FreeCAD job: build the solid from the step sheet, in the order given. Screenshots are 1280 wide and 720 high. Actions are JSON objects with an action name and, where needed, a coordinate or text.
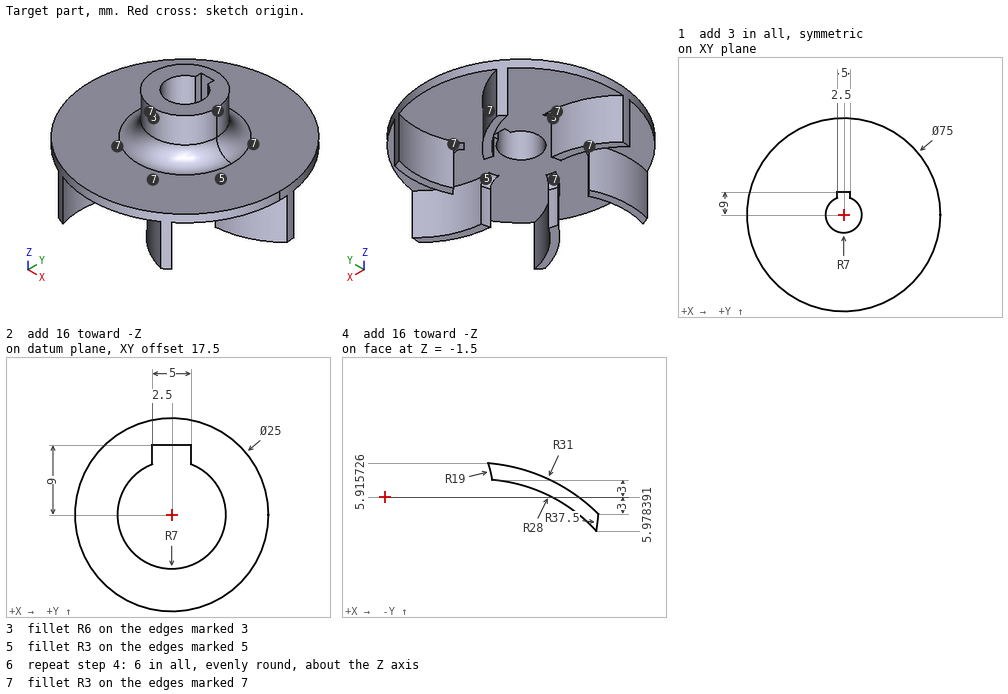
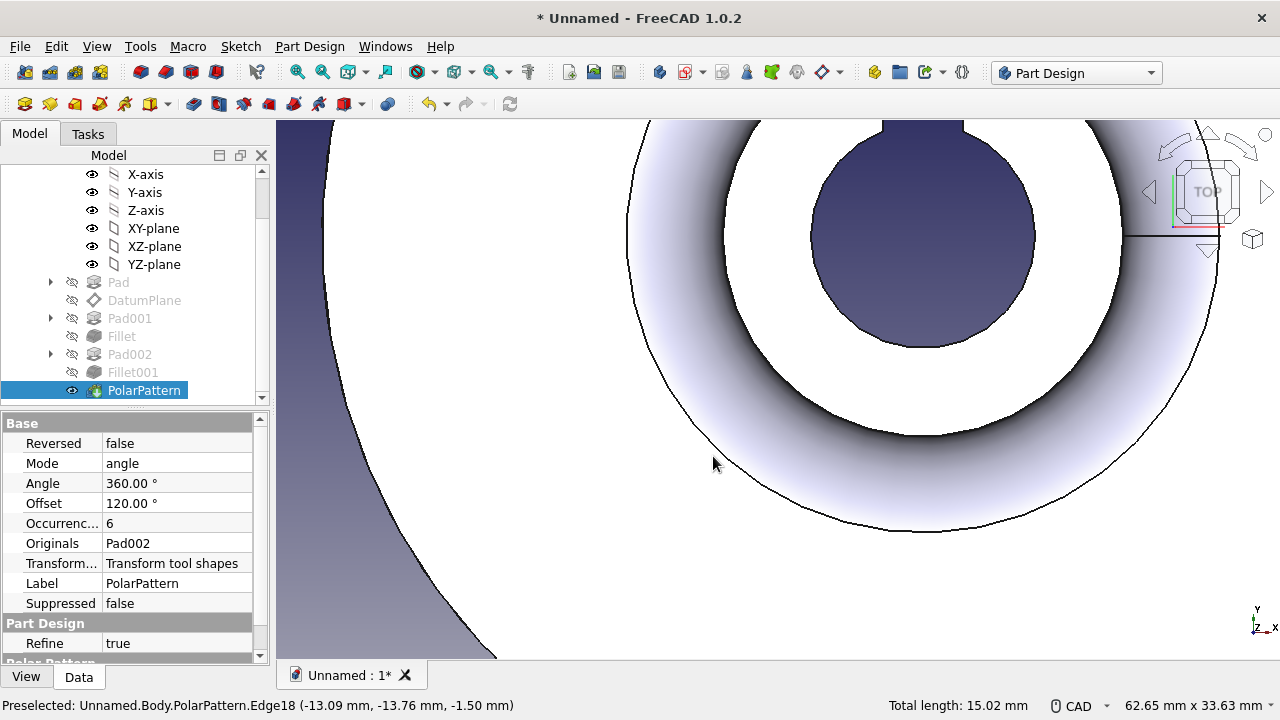
{"action": "left_click", "coordinate": [141, 72]}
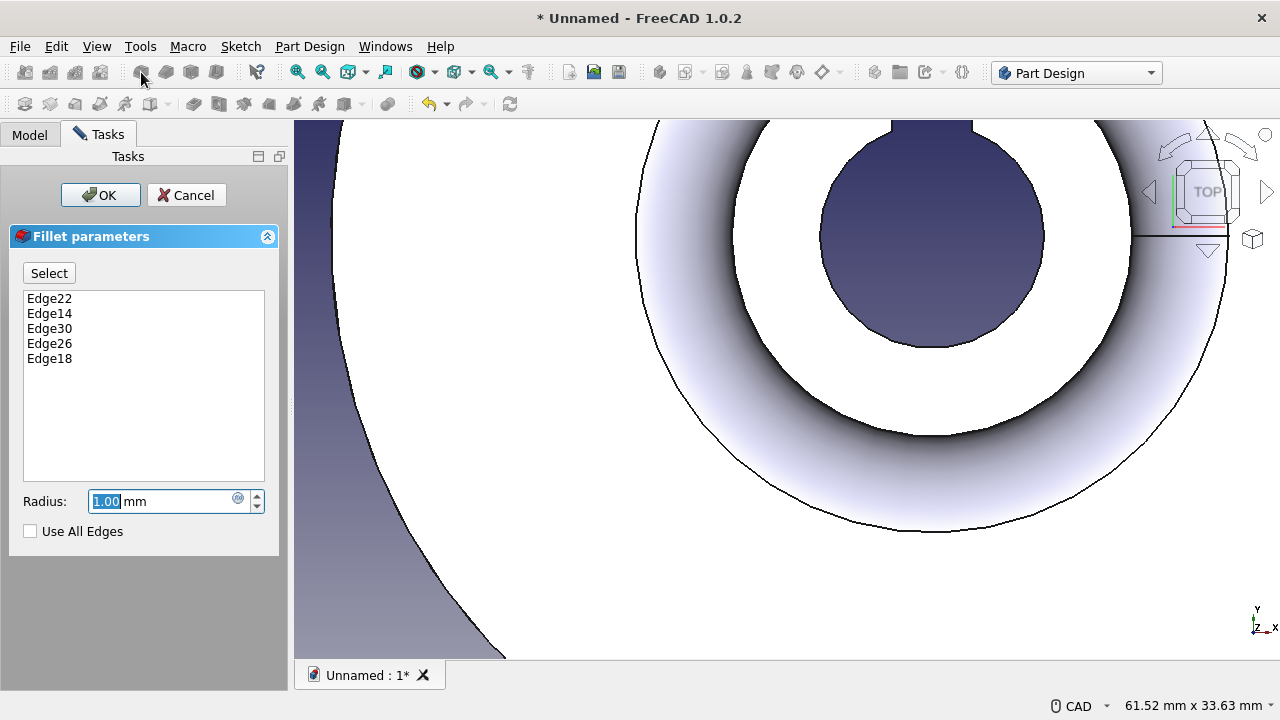
{"action": "type", "text": "3"}
{"action": "key", "text": "Tab"}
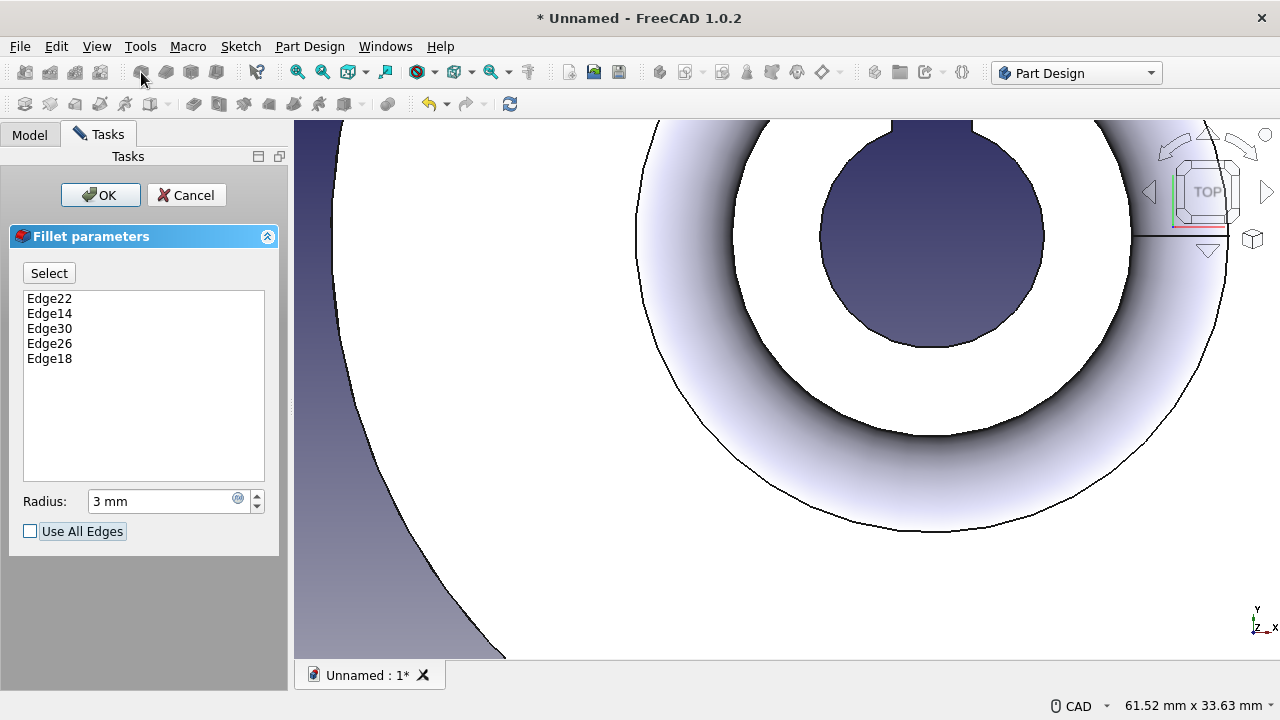
{"action": "left_click", "coordinate": [101, 195]}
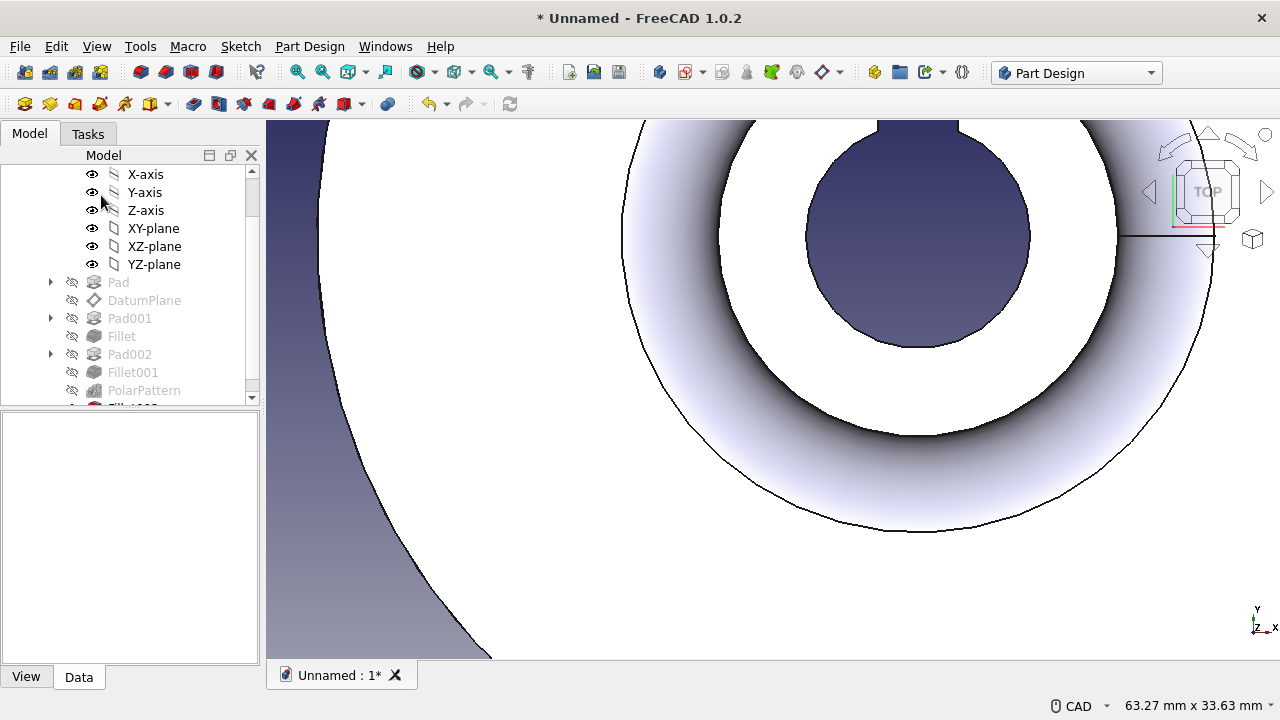
{"action": "key", "text": "0"}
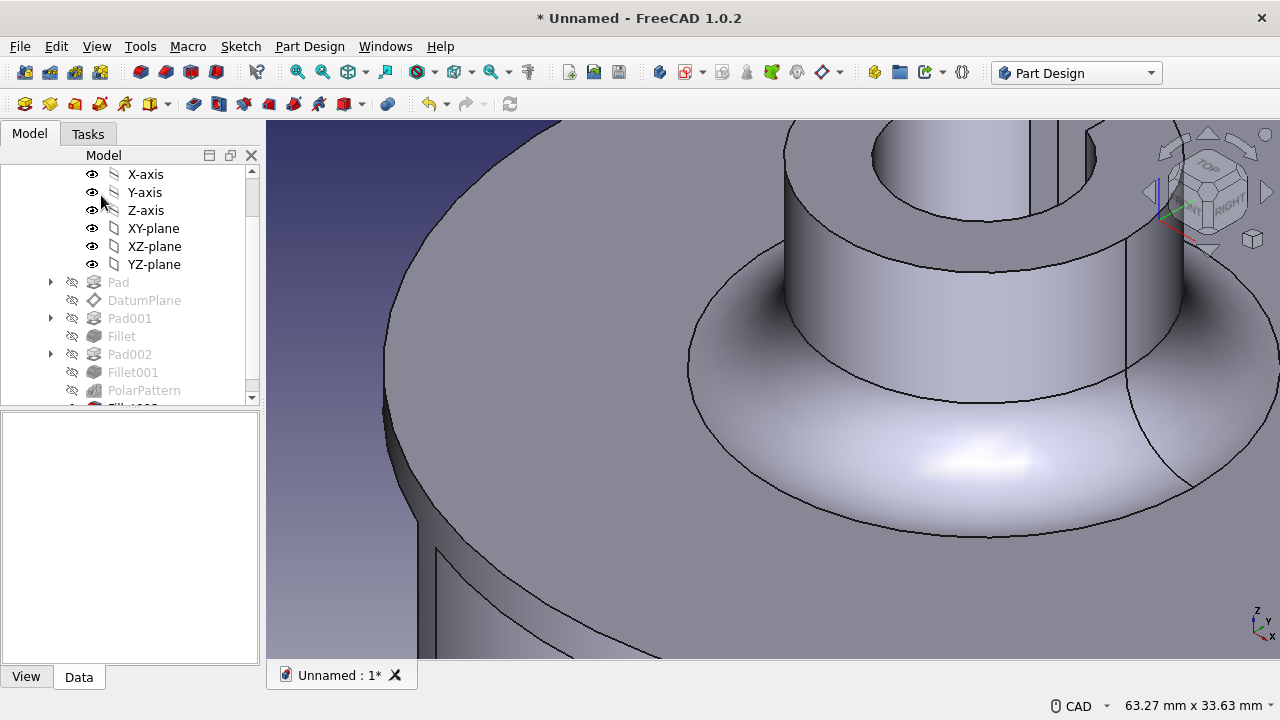
{"action": "left_click", "coordinate": [298, 72]}